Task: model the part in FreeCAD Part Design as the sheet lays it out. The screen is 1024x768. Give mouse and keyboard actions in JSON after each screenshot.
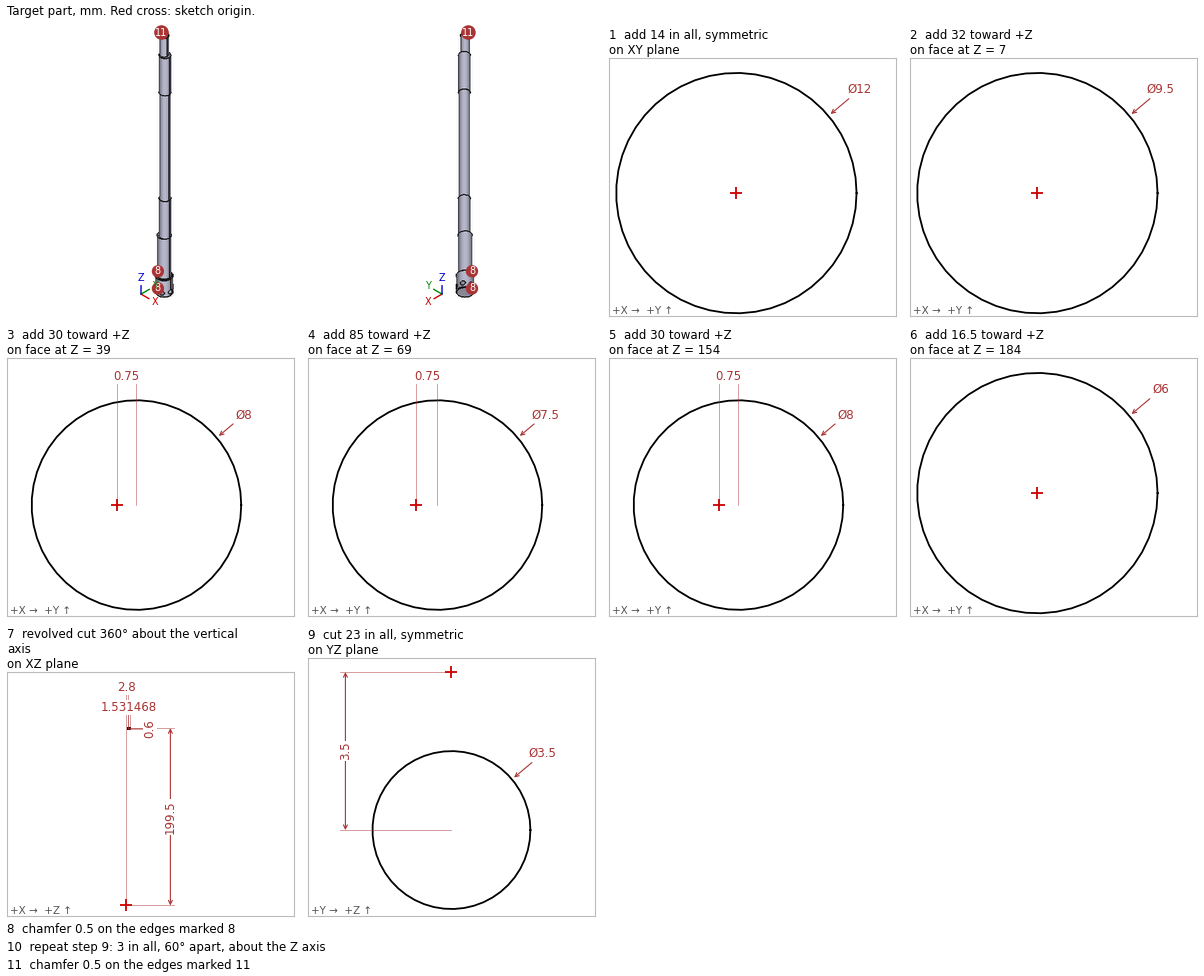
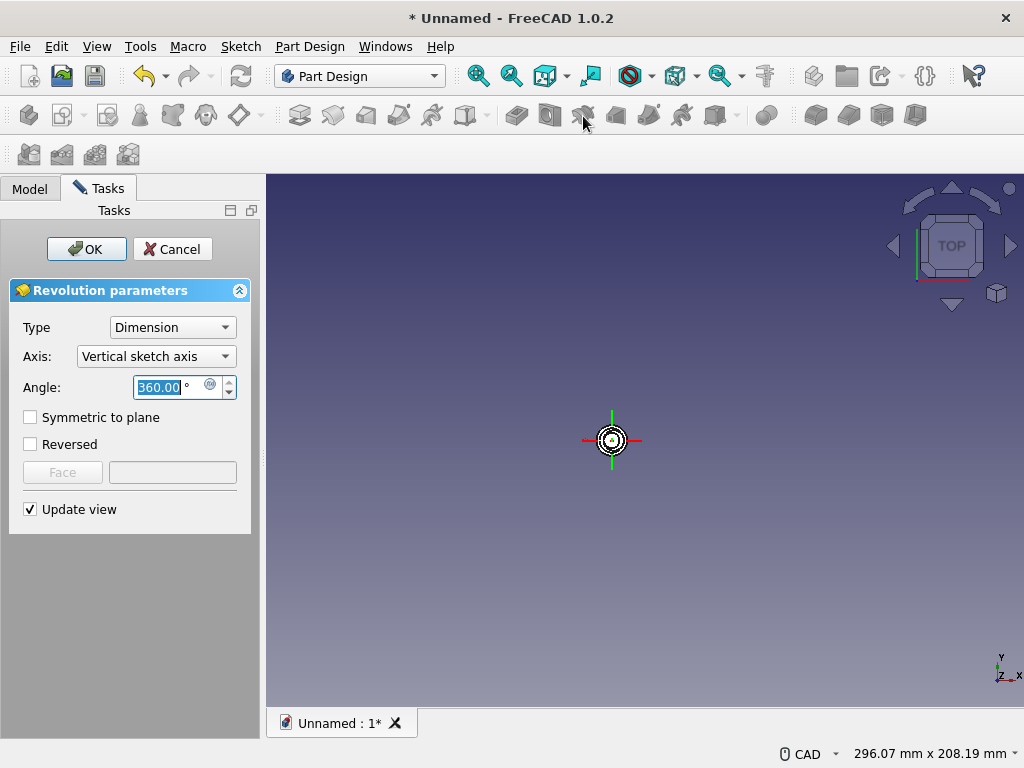
{"action": "left_click", "coordinate": [87, 249]}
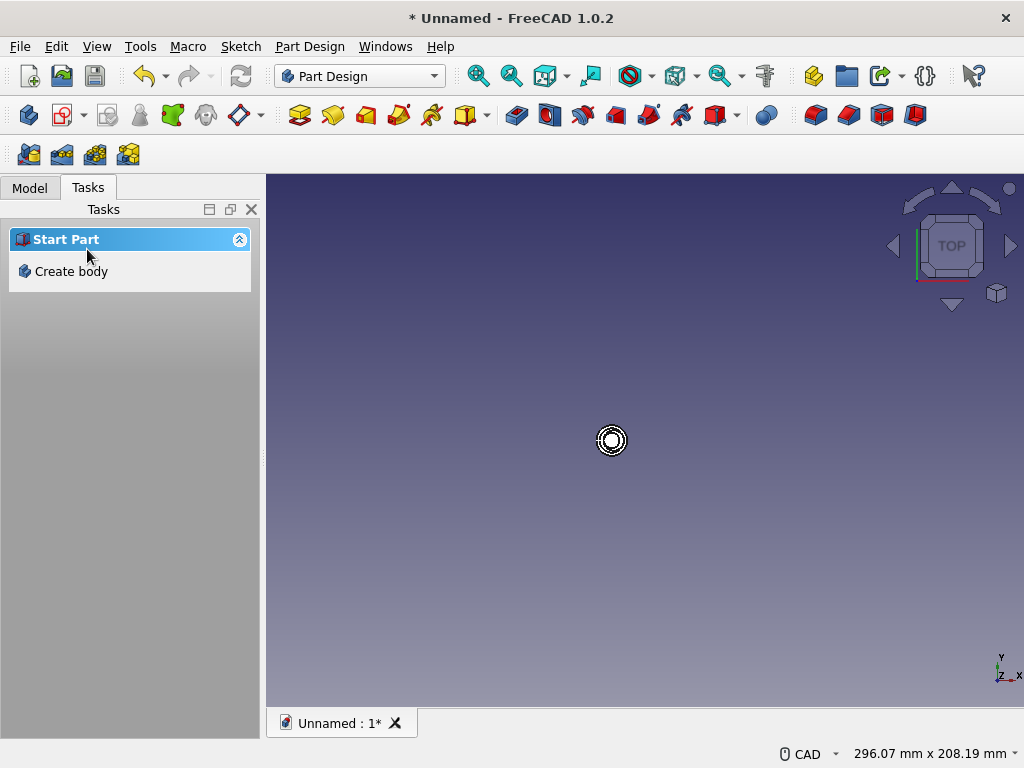
{"action": "key", "text": "v f"}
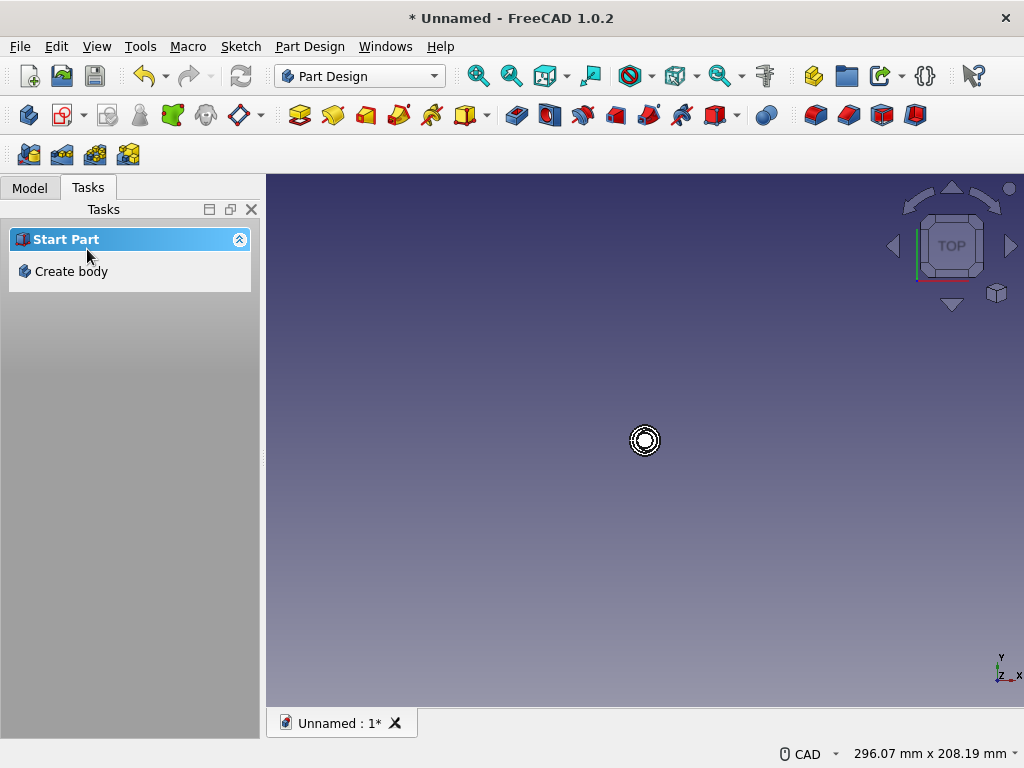
{"action": "key", "text": "0"}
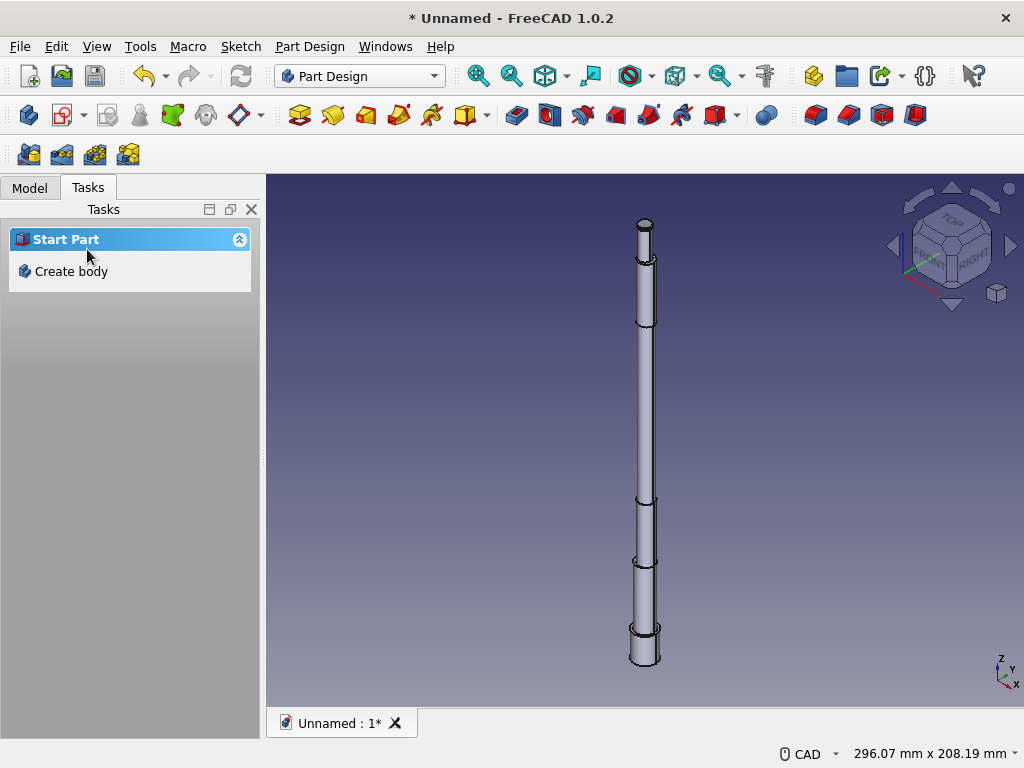
{"action": "left_click", "coordinate": [631, 631]}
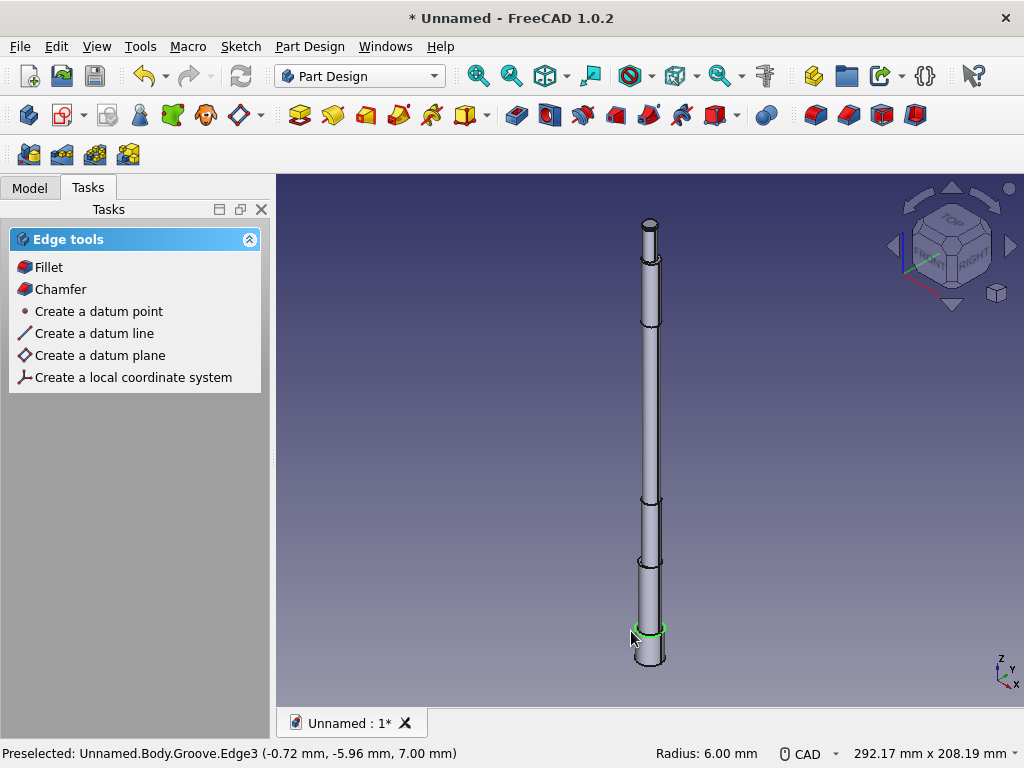
{"action": "key", "text": "2"}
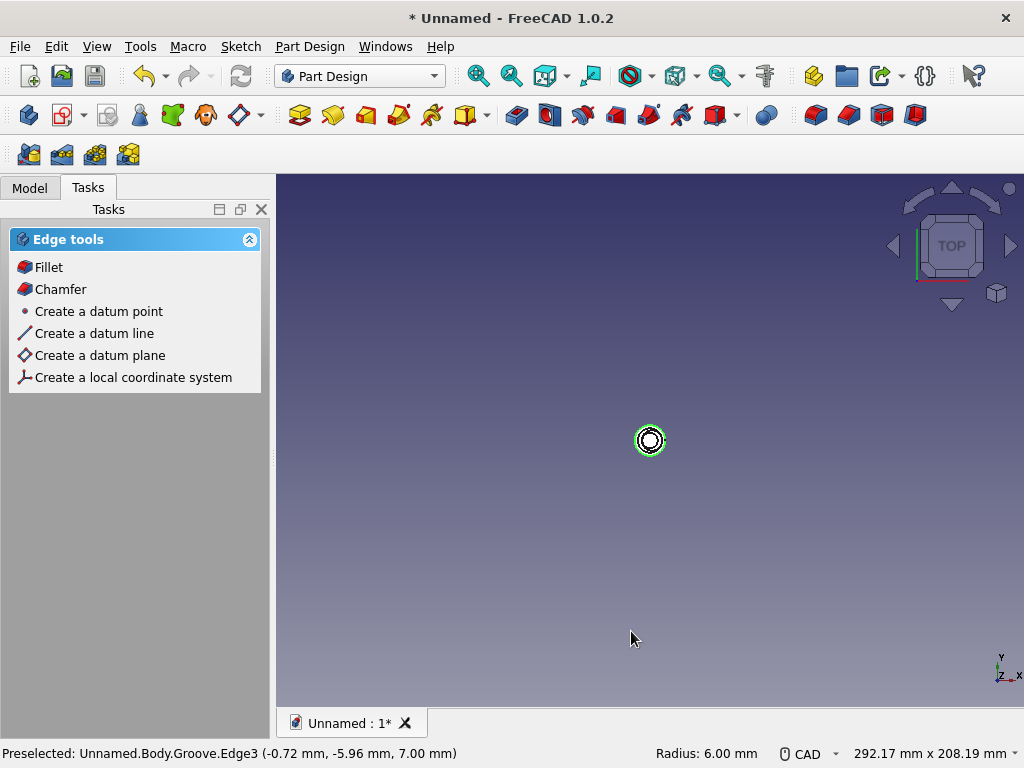
{"action": "left_click", "coordinate": [479, 76]}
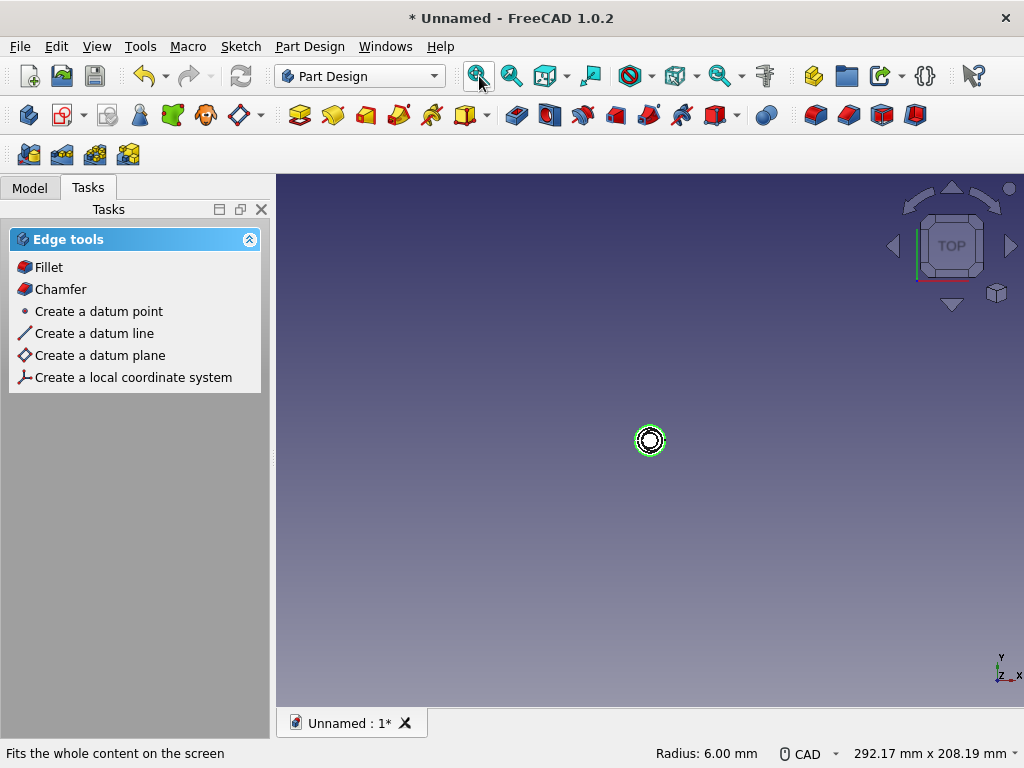
{"action": "key", "text": "1"}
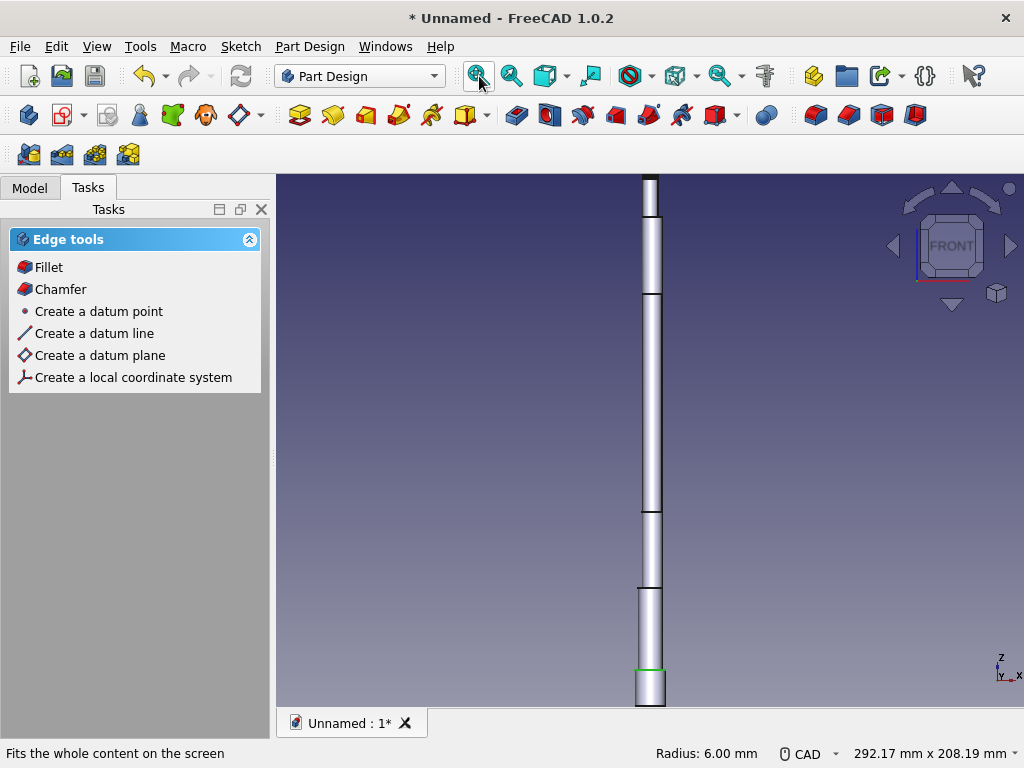
{"action": "key", "text": "3"}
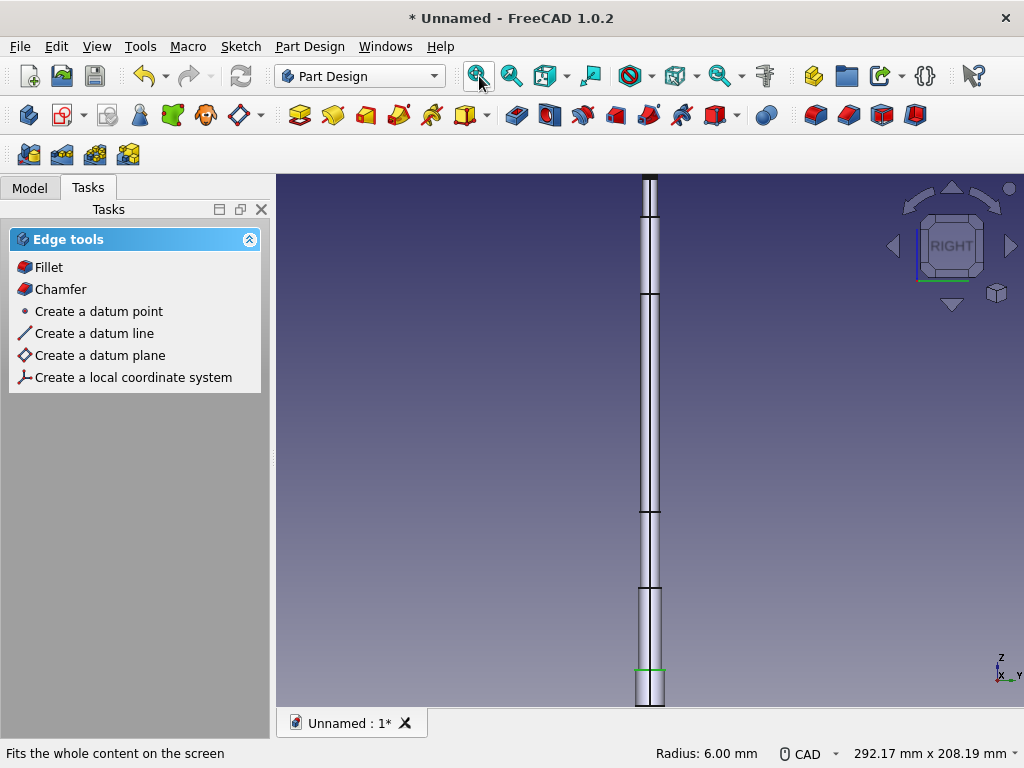
{"action": "key", "text": "5"}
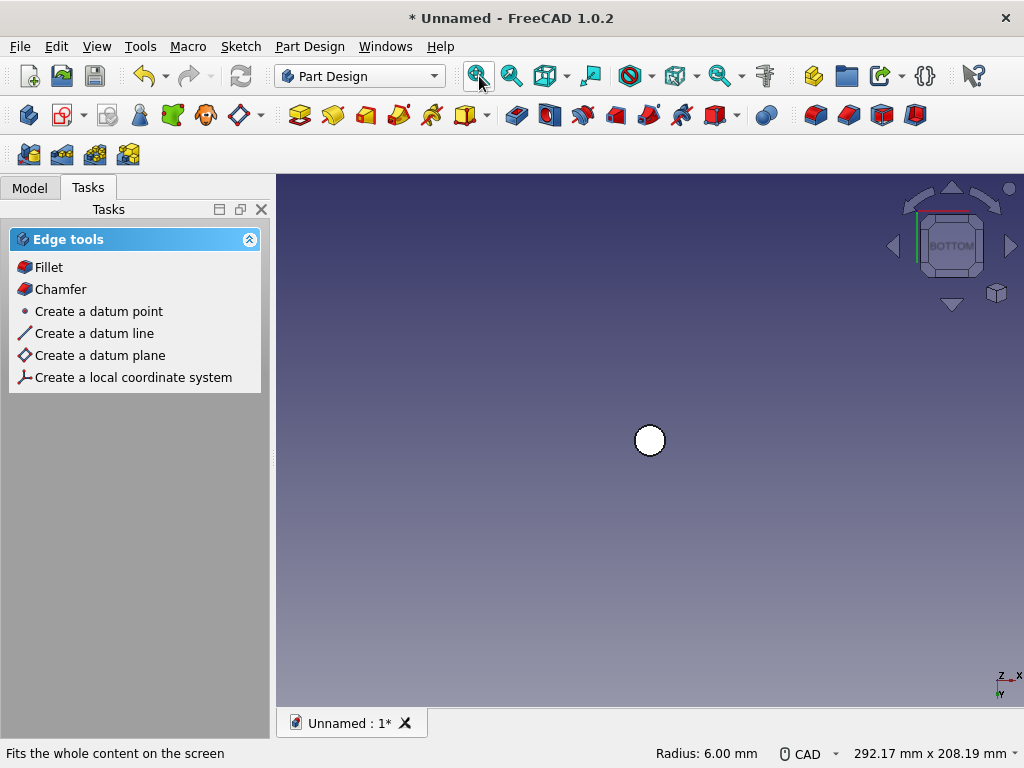
{"action": "key", "text": "v f"}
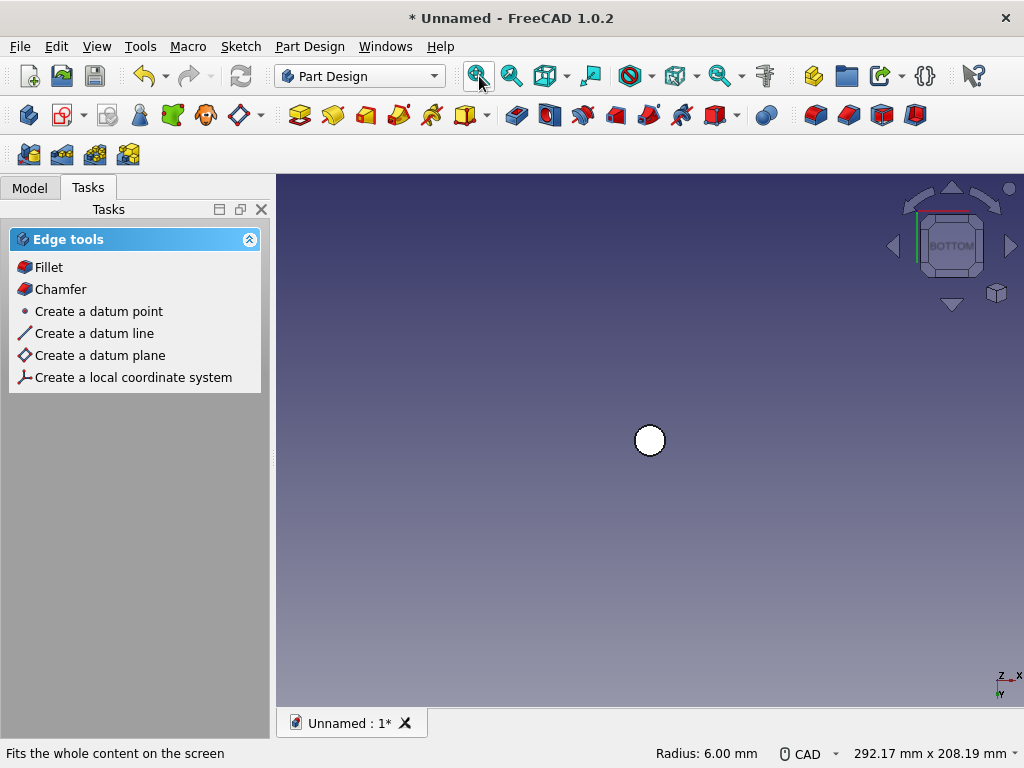
{"action": "left_click", "coordinate": [635, 439], "text": "ctrl"}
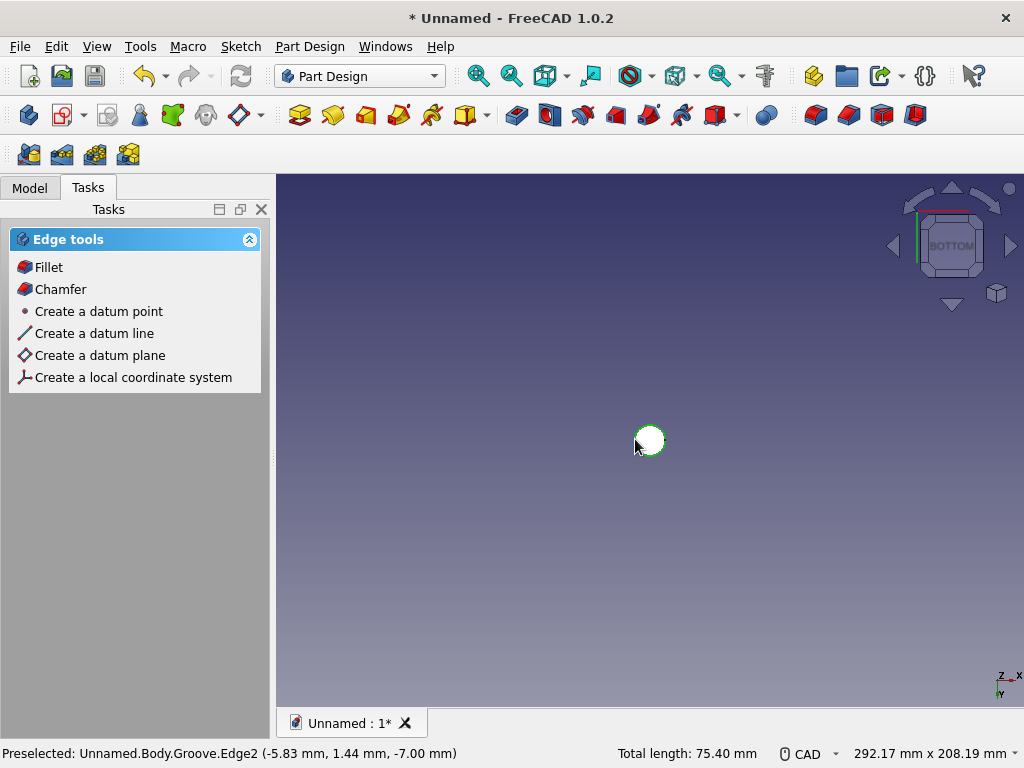
{"action": "left_click", "coordinate": [849, 116]}